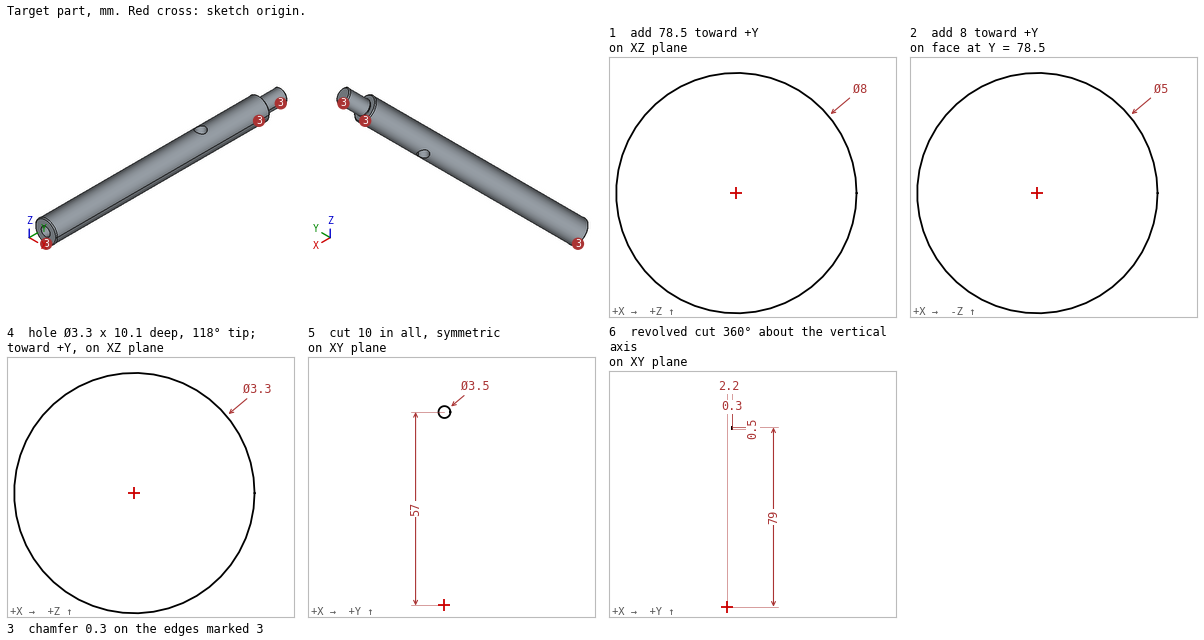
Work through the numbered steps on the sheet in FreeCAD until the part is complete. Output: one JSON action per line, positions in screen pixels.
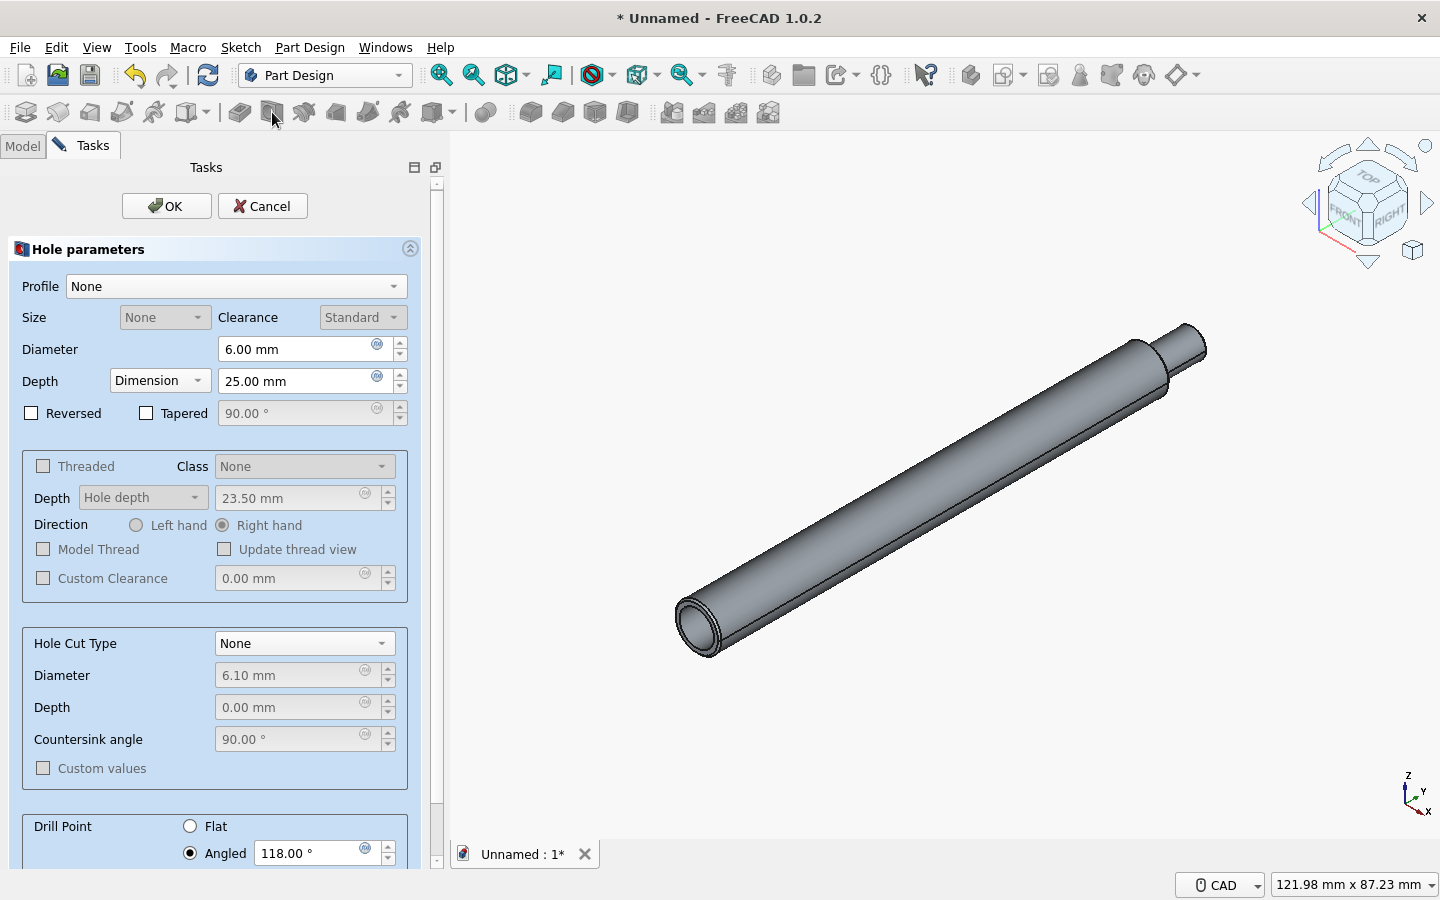
{"action": "triple_click", "coordinate": [305, 349]}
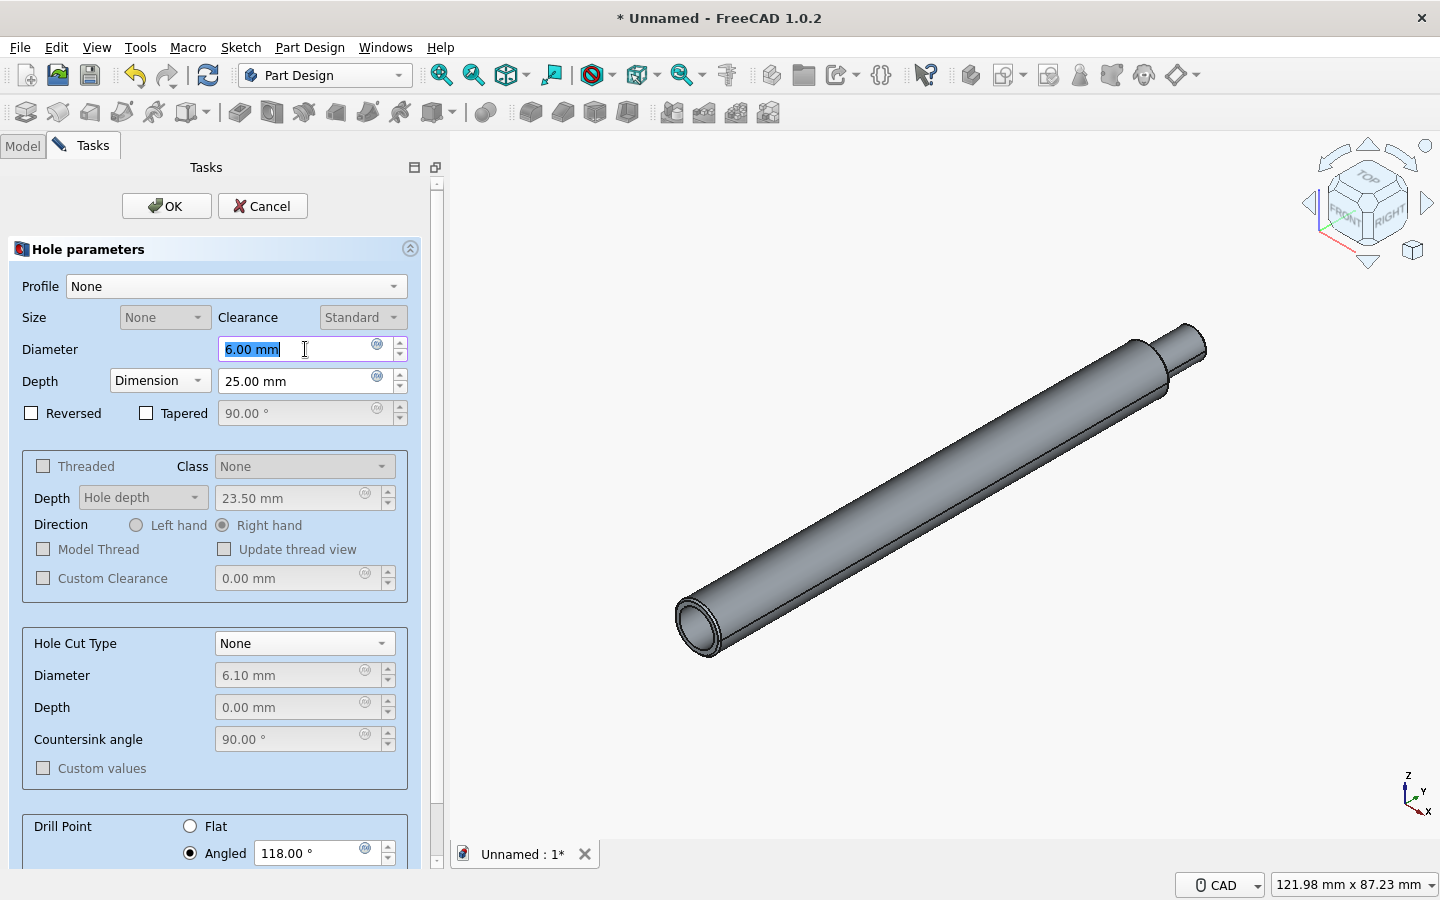
{"action": "type", "text": "3.3"}
{"action": "key", "text": "Tab"}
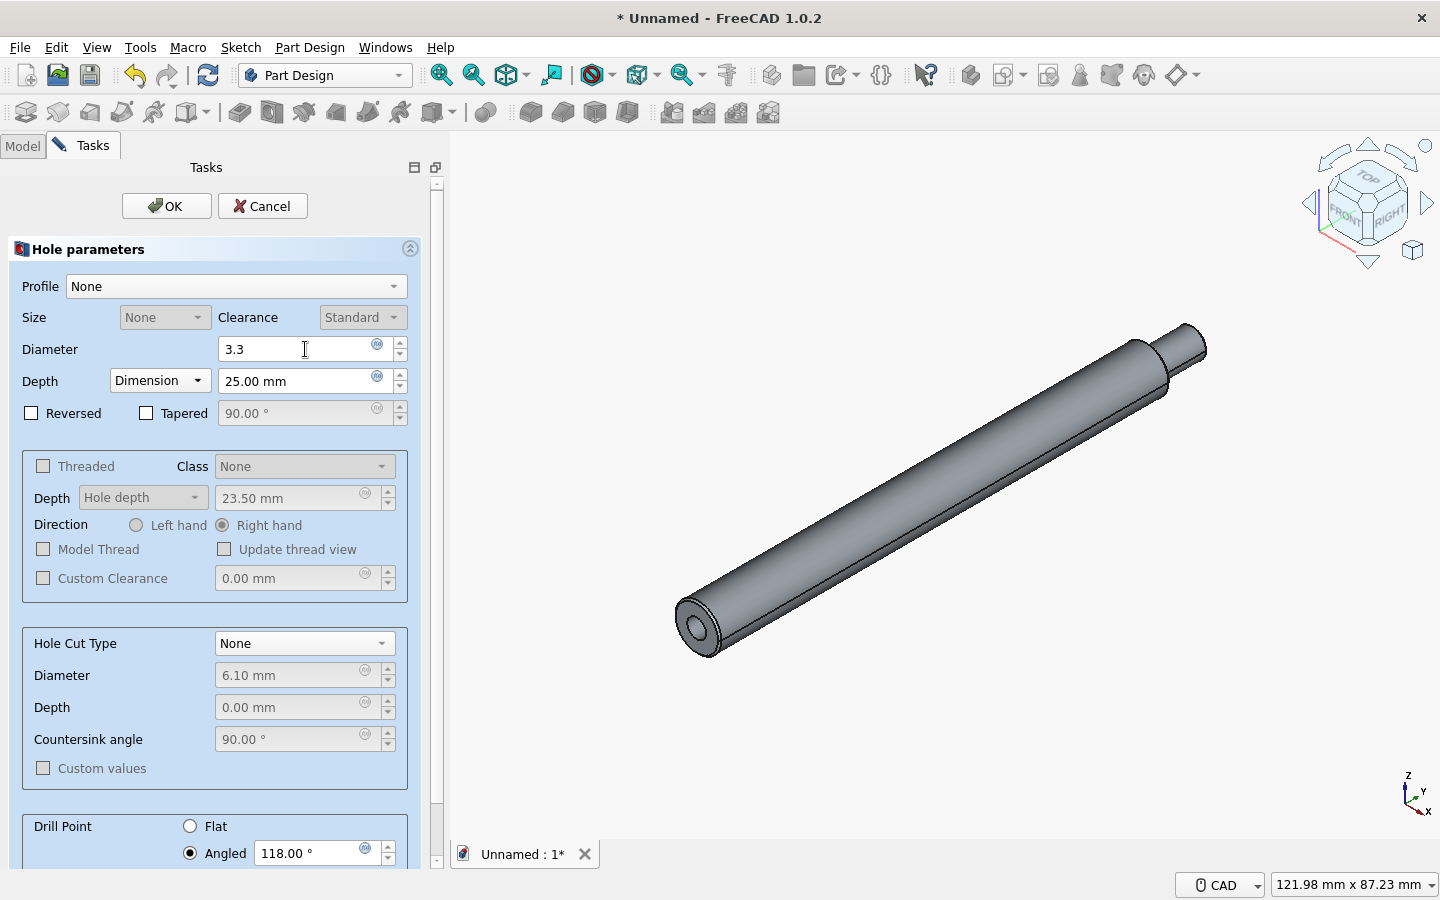
{"action": "triple_click", "coordinate": [305, 381]}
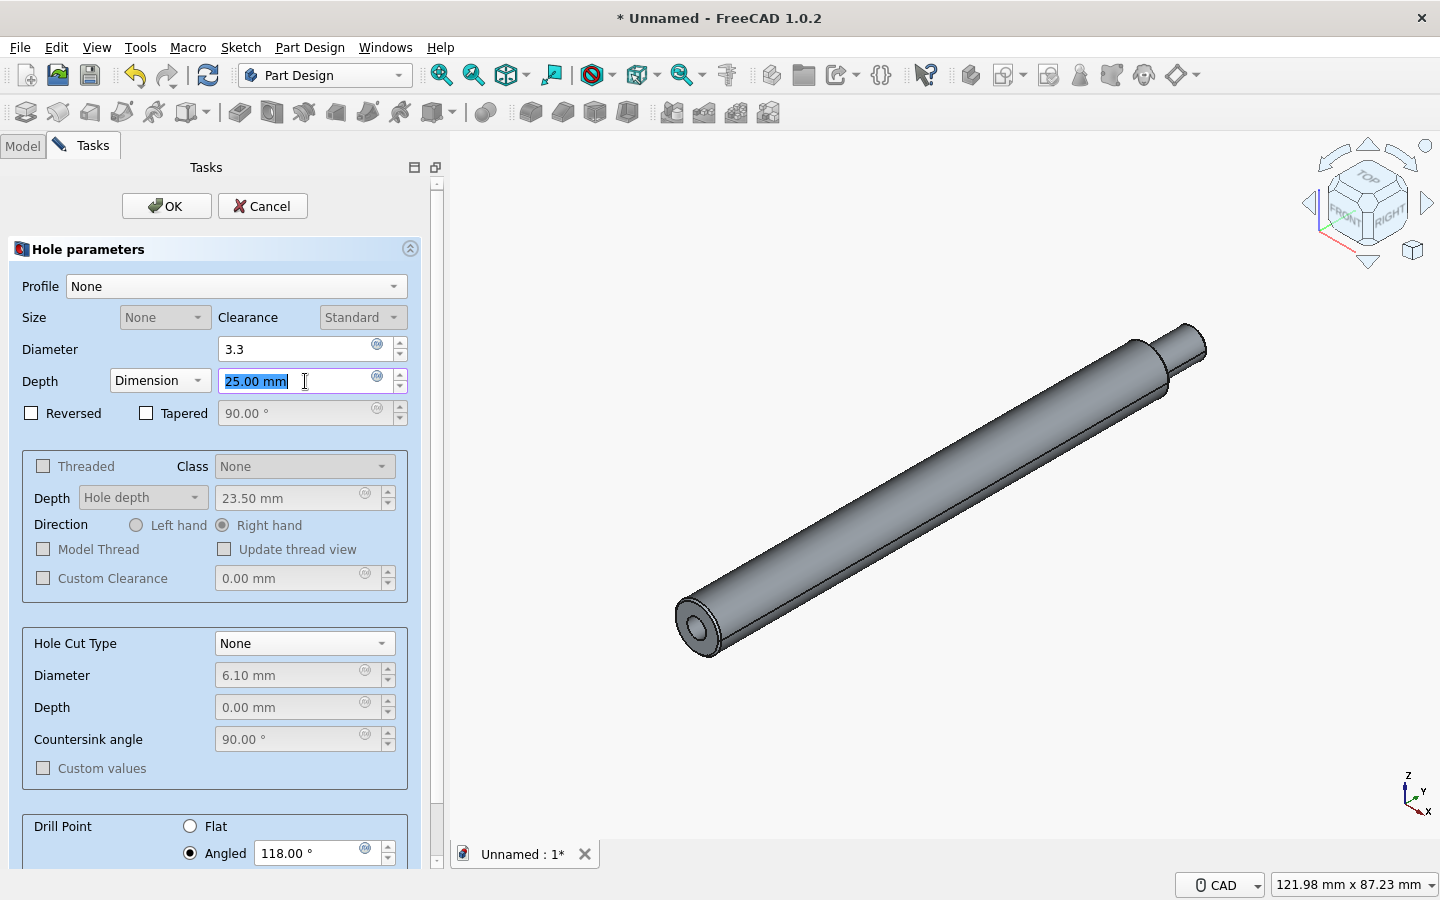
{"action": "type", "text": "10.1"}
{"action": "key", "text": "Tab"}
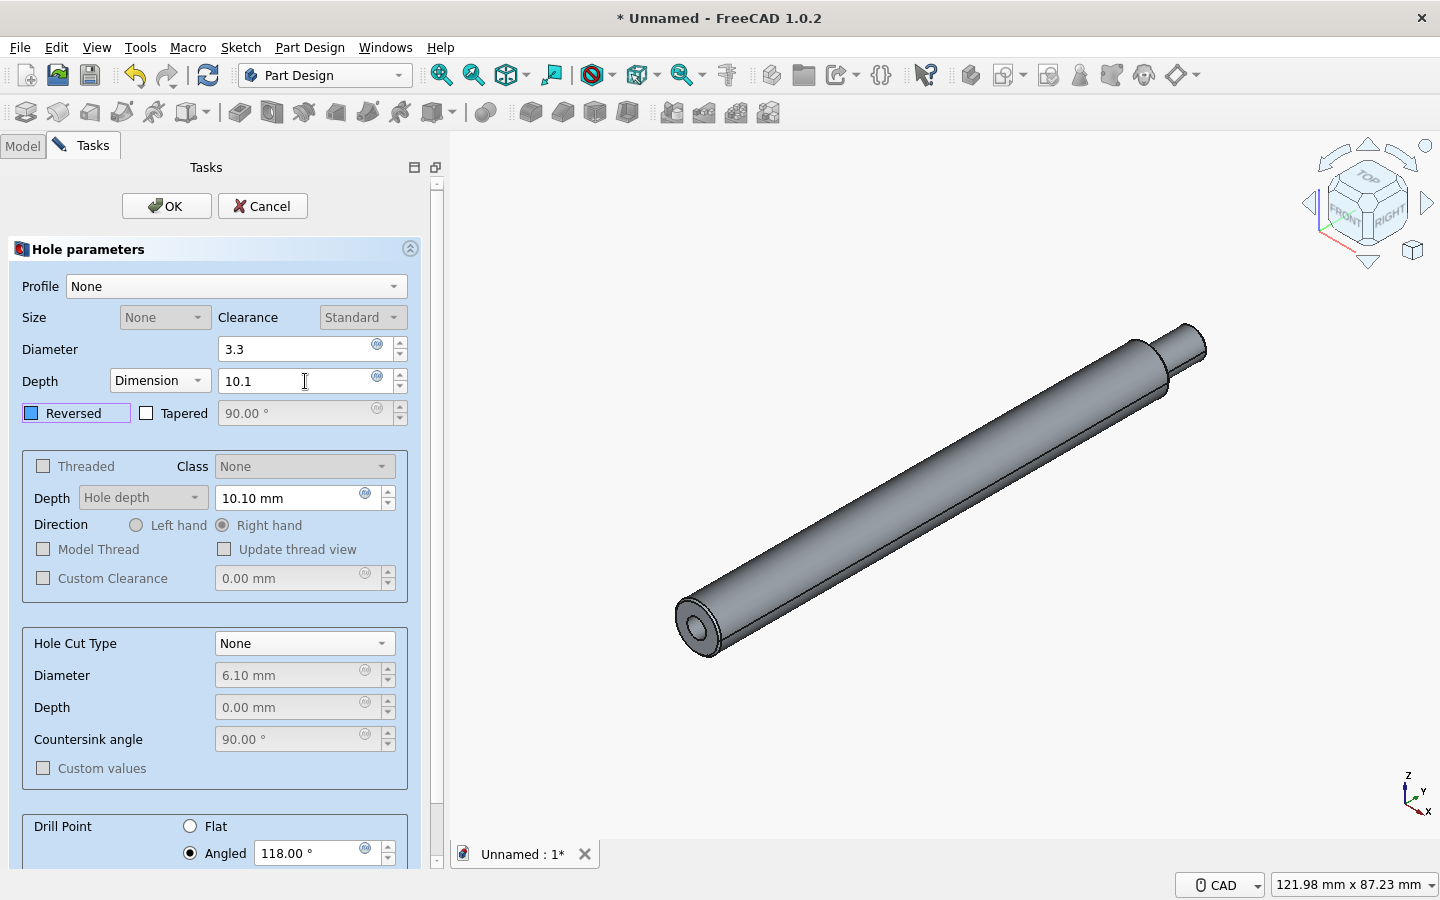
{"action": "left_click", "coordinate": [167, 206]}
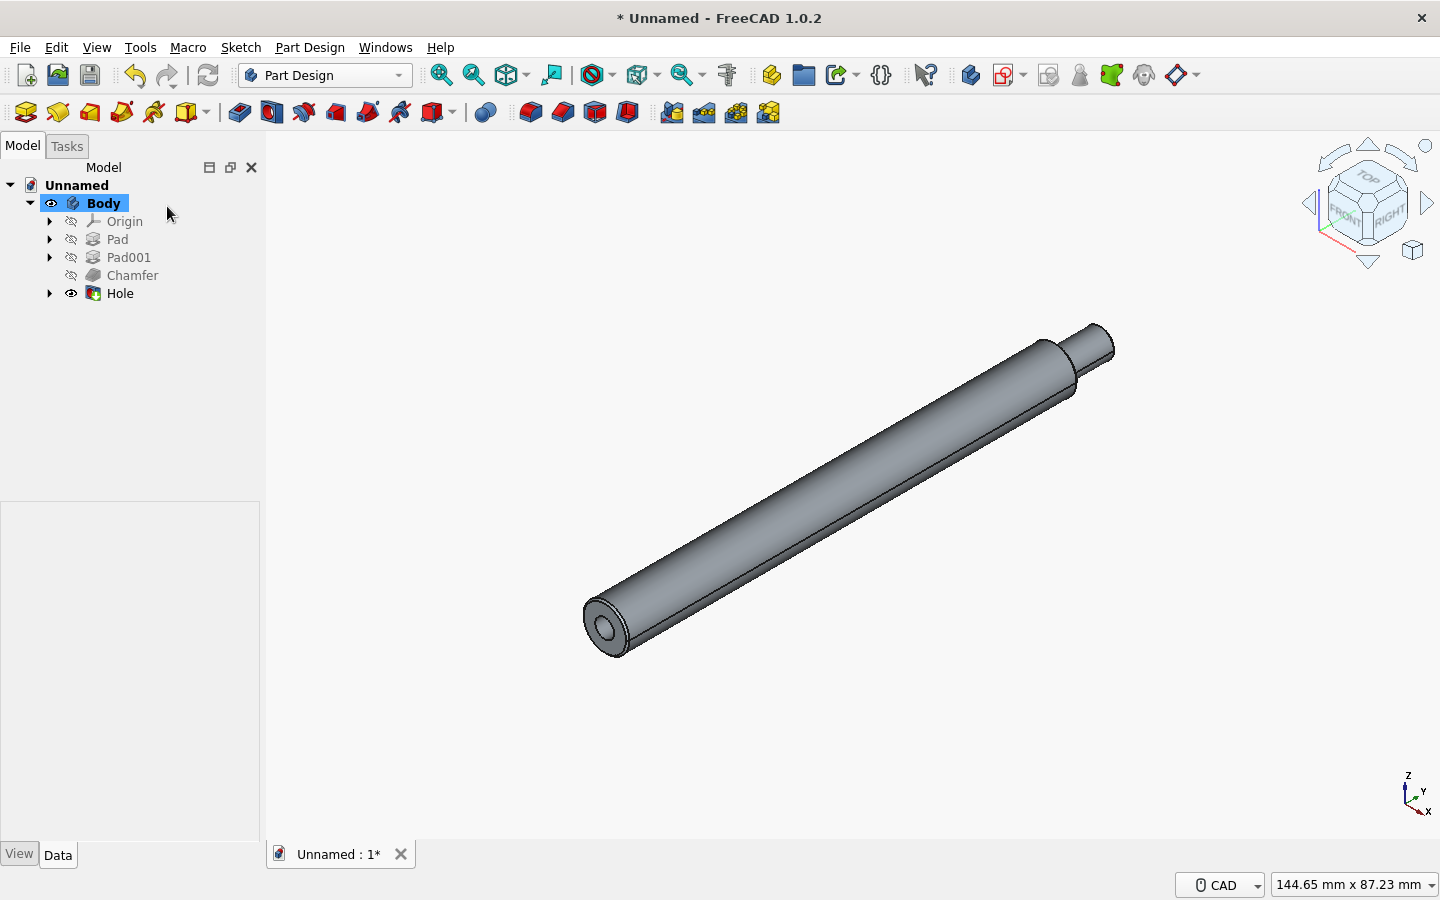
{"action": "left_click", "coordinate": [1004, 76]}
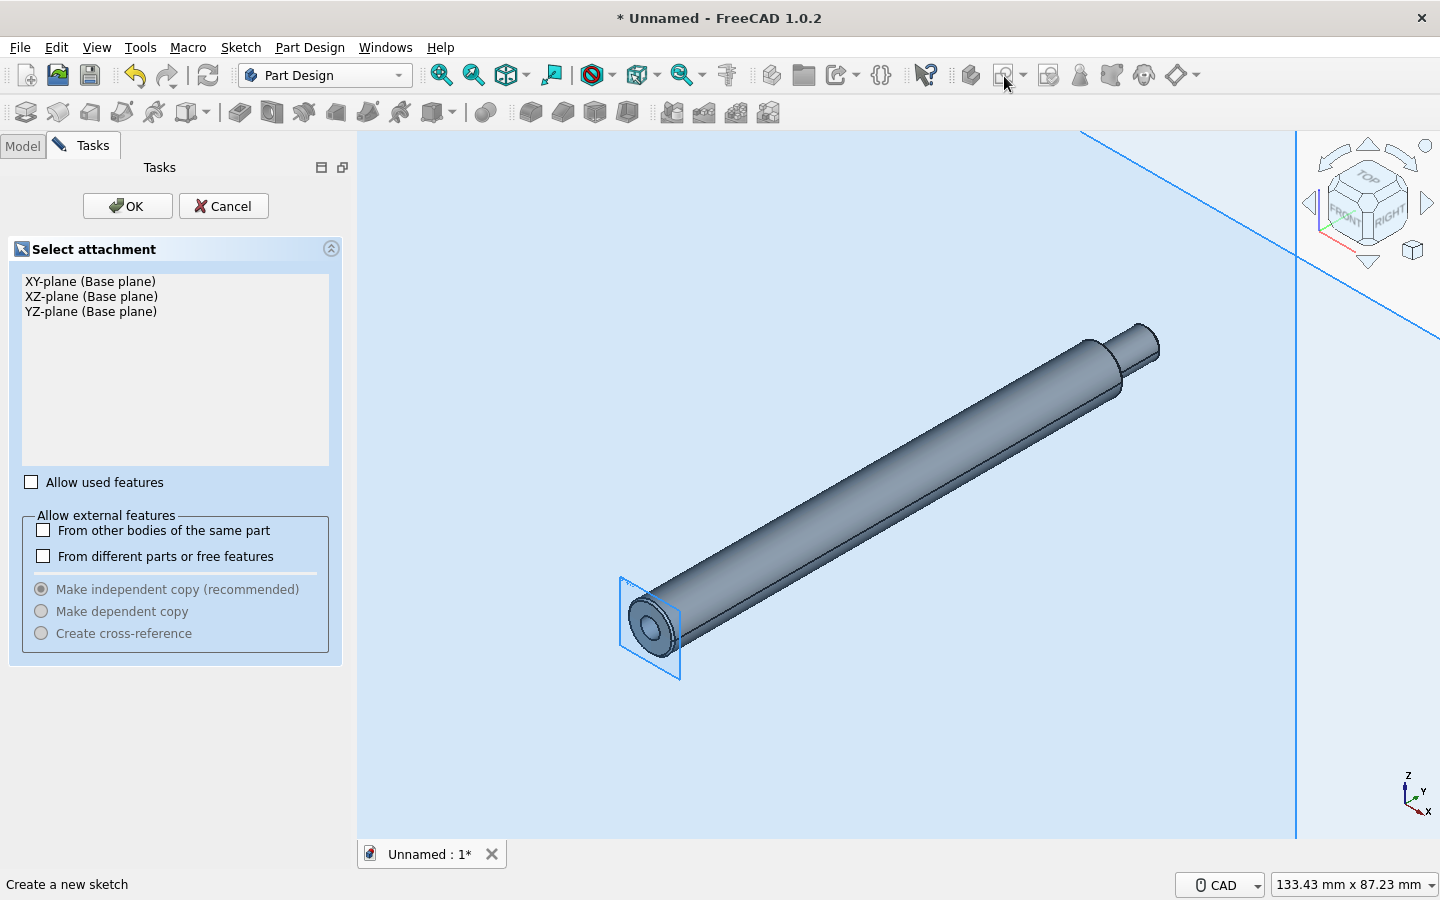
{"action": "left_click", "coordinate": [82, 282]}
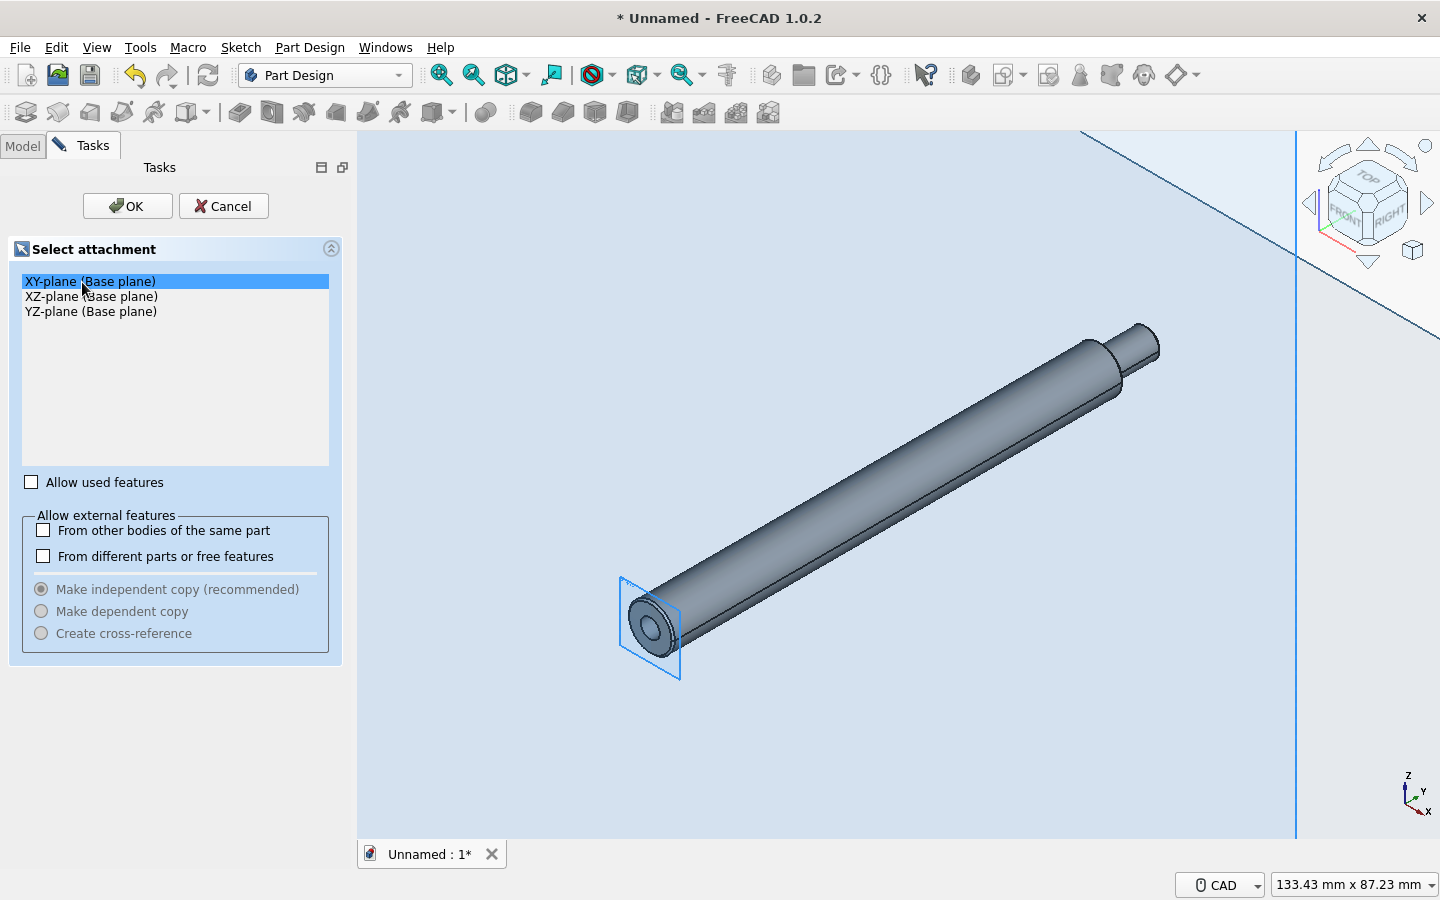
{"action": "left_click", "coordinate": [128, 206]}